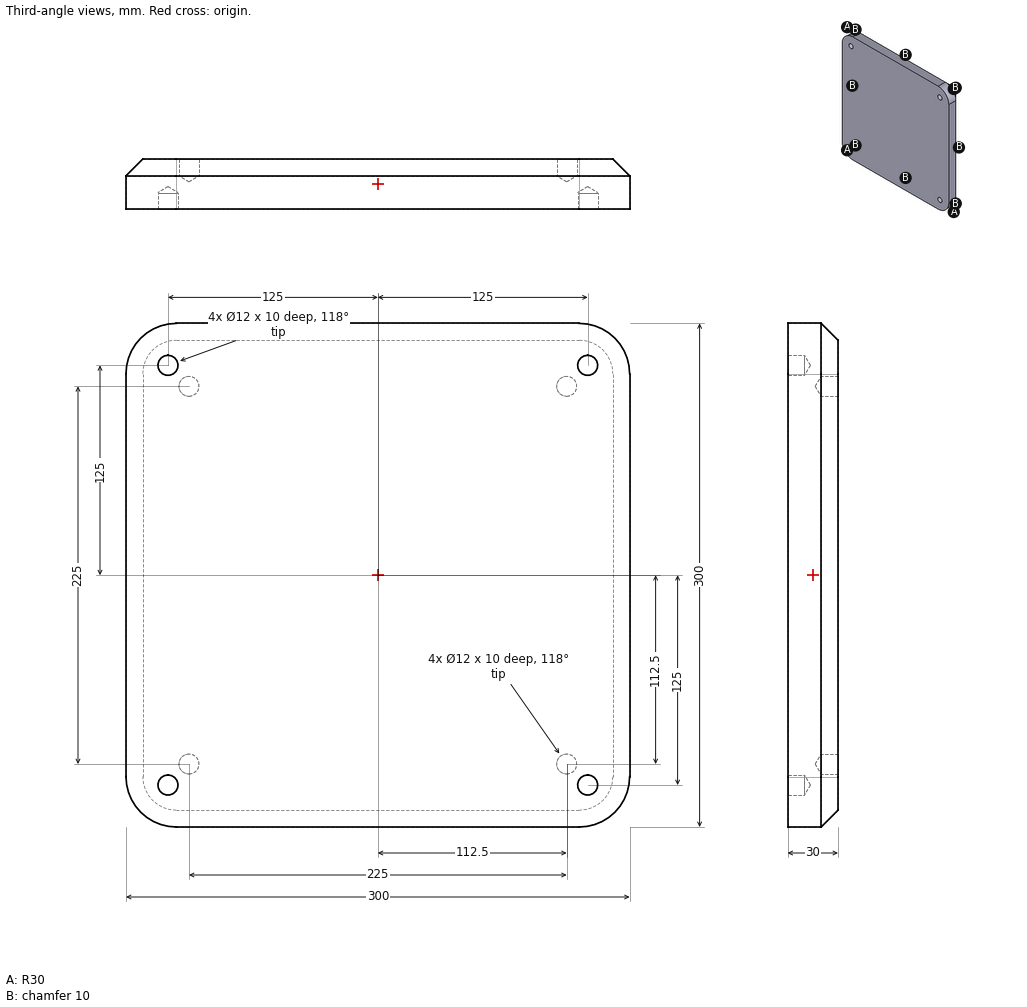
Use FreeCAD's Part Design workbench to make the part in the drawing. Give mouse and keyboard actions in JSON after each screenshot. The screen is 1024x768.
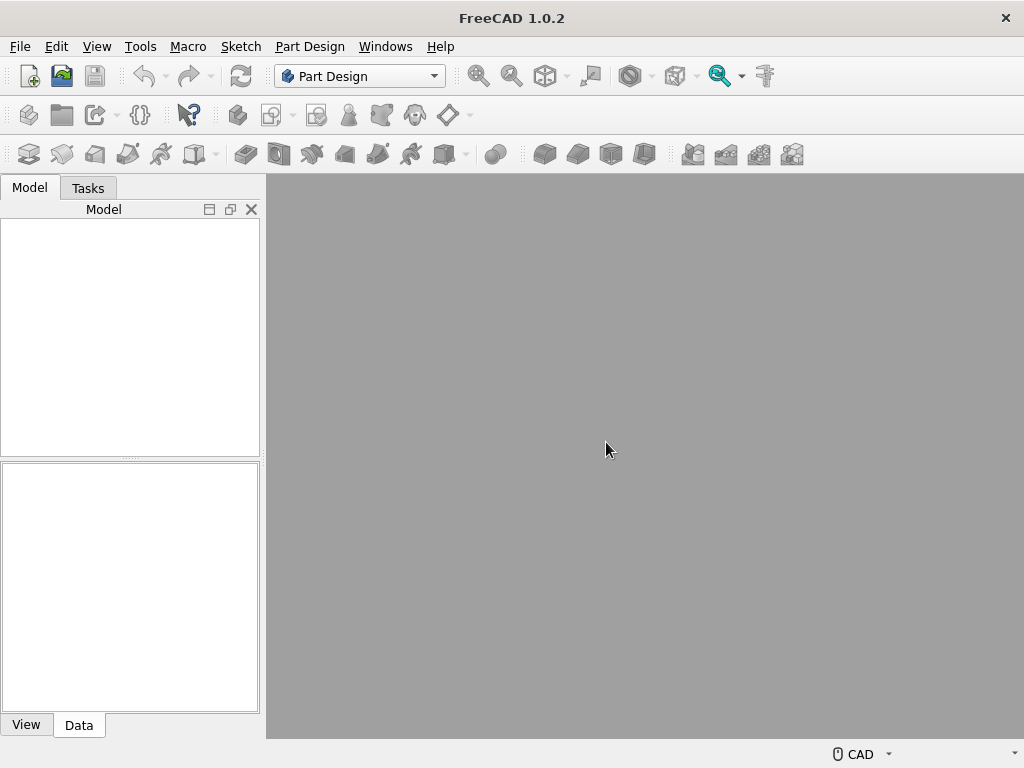
{"action": "left_click", "coordinate": [29, 76]}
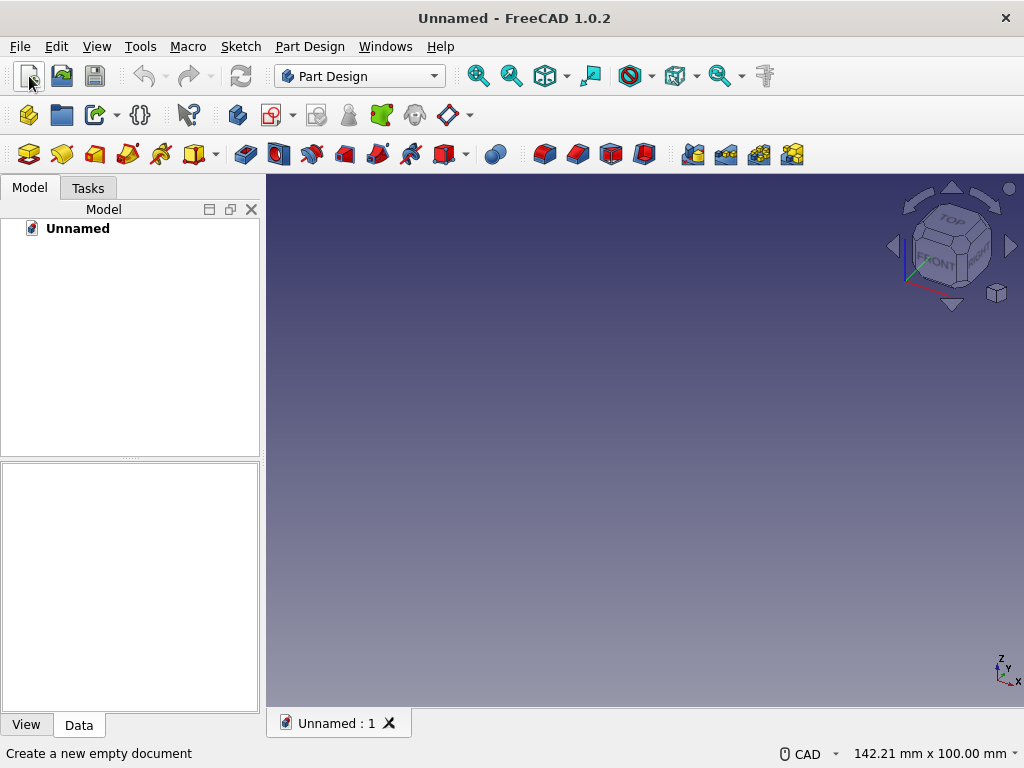
{"action": "left_click", "coordinate": [270, 116]}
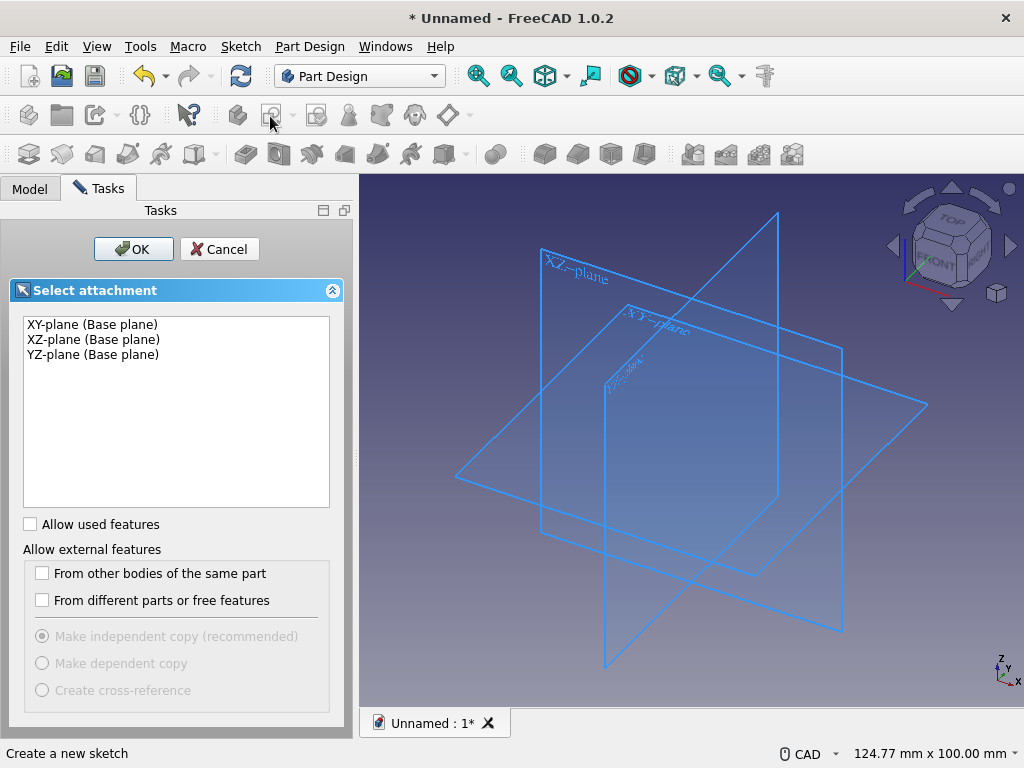
{"action": "left_click", "coordinate": [84, 340]}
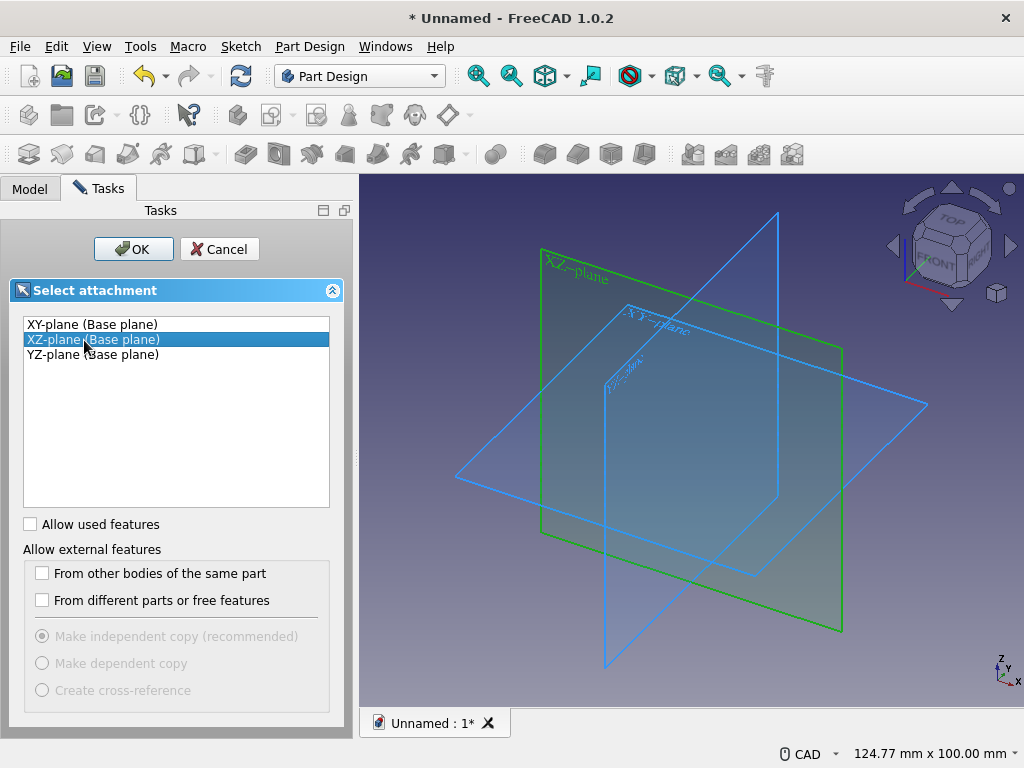
{"action": "left_click", "coordinate": [134, 249]}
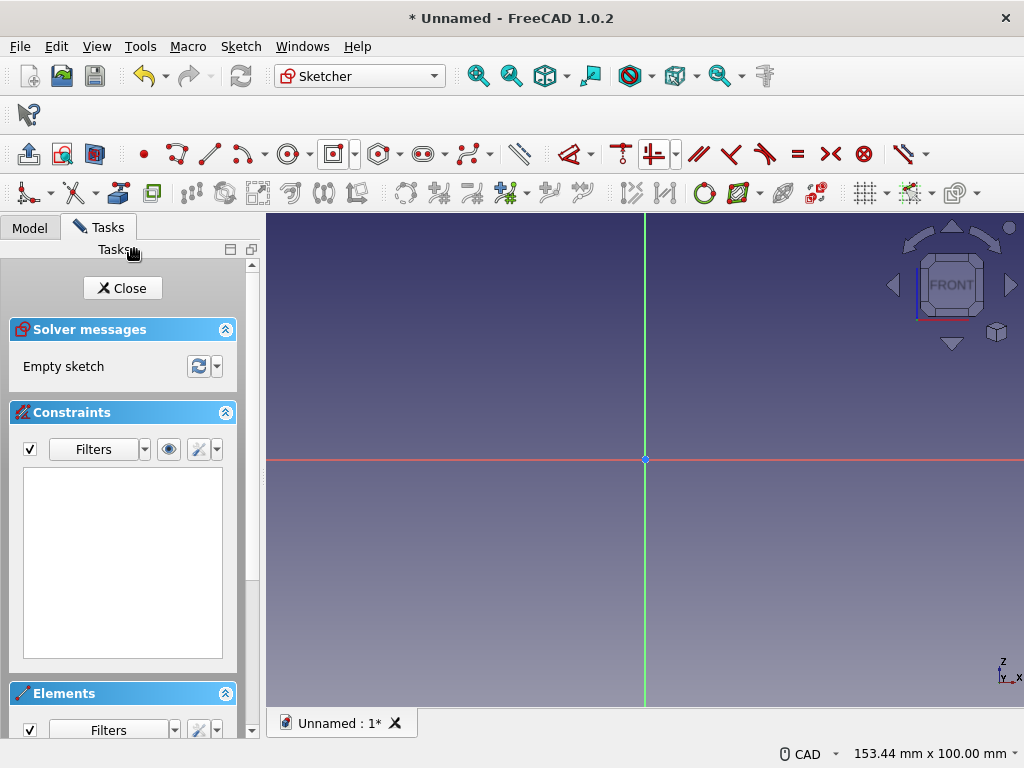
{"action": "scroll", "coordinate": [559, 460], "scroll_direction": "down", "scroll_amount": 8}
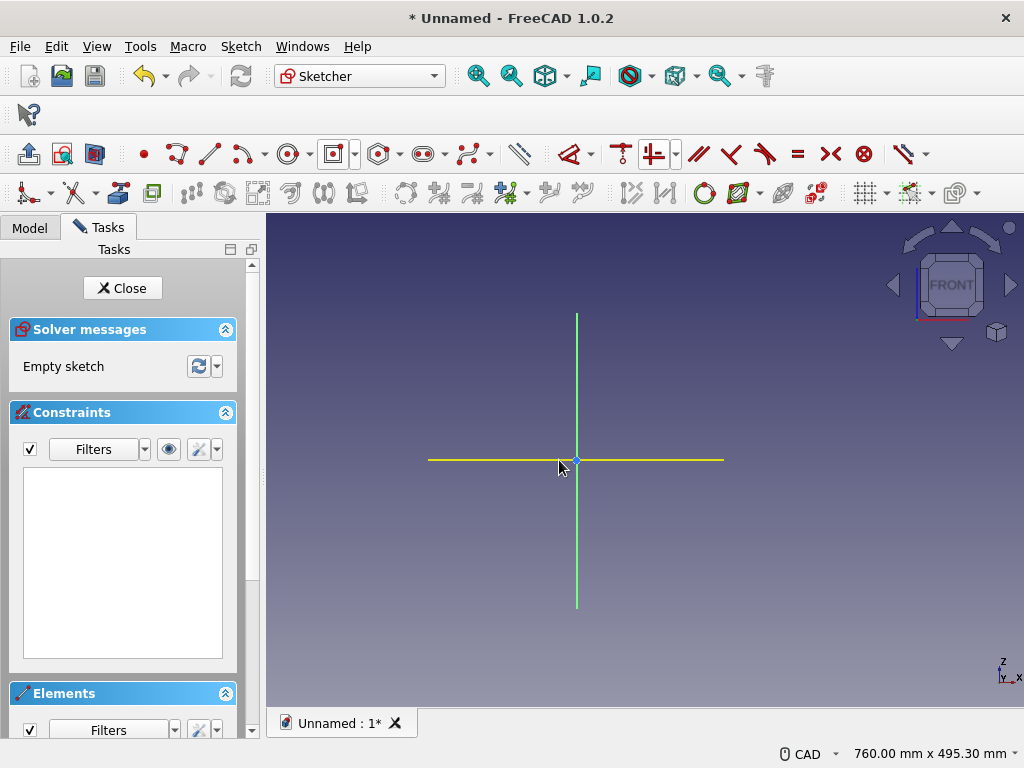
{"action": "left_click", "coordinate": [332, 154]}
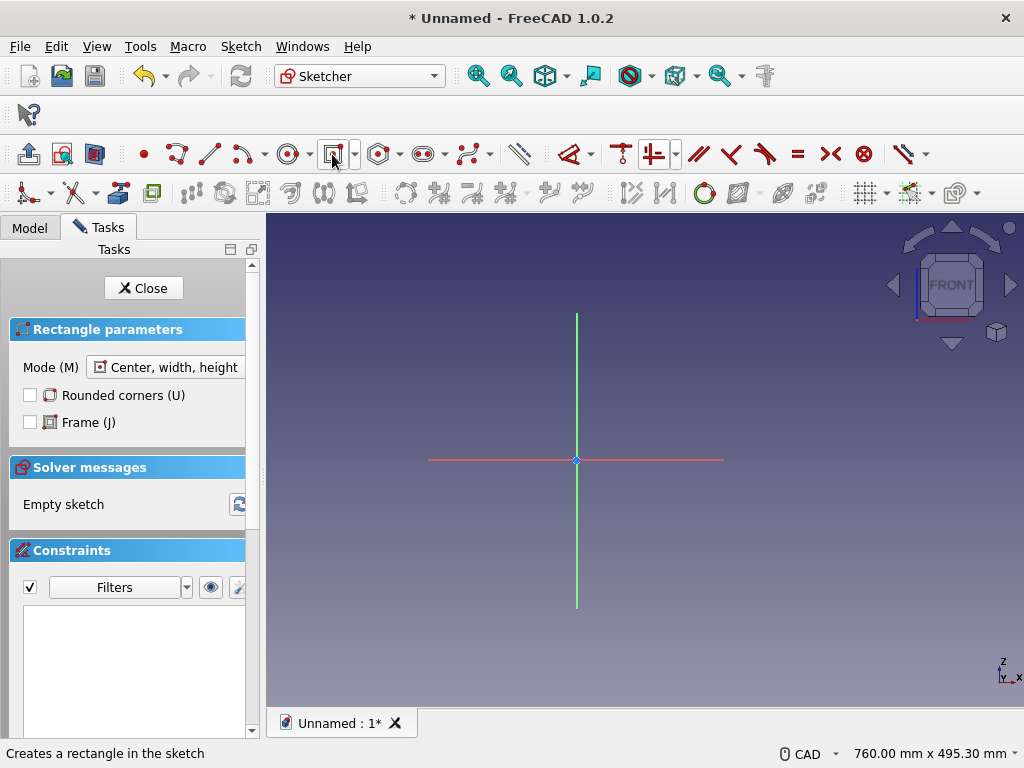
{"action": "left_click", "coordinate": [577, 460]}
{"action": "left_click", "coordinate": [726, 311]}
{"action": "key", "text": "Escape"}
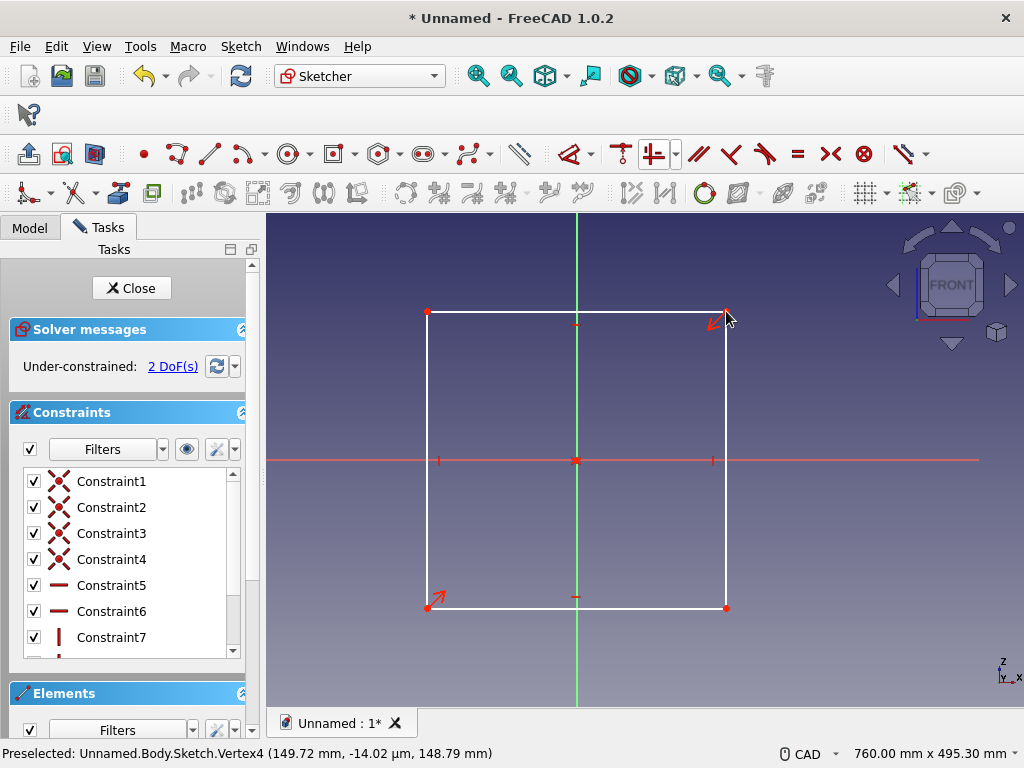
{"action": "left_click", "coordinate": [568, 154]}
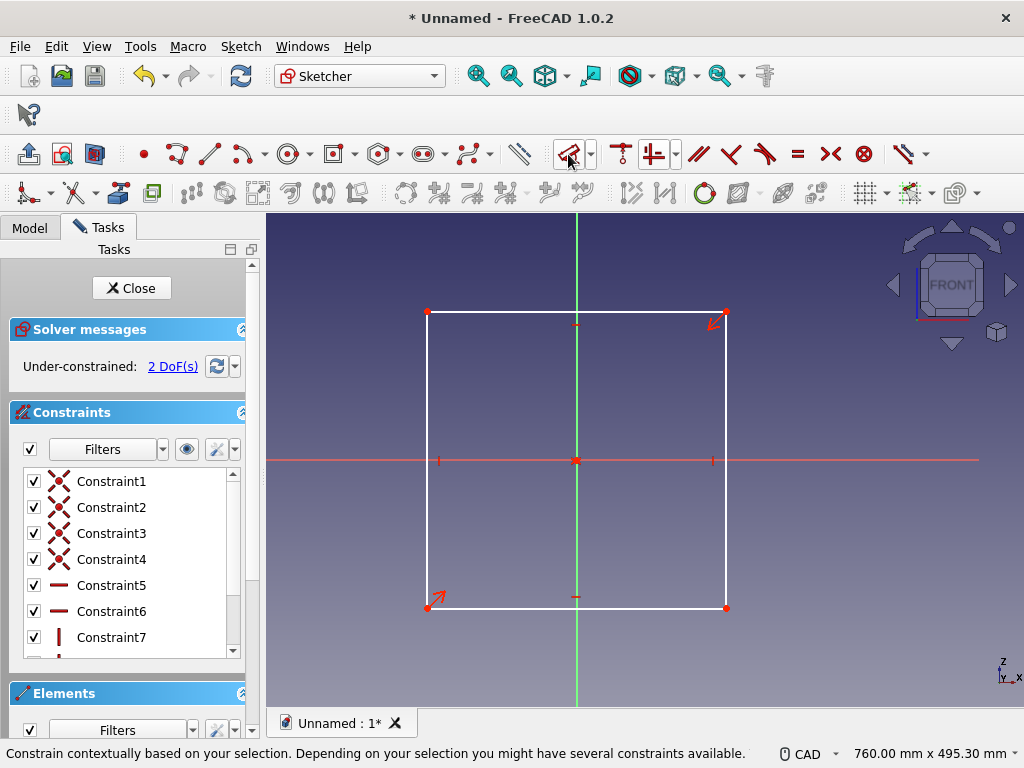
{"action": "left_click", "coordinate": [517, 609]}
{"action": "left_click", "coordinate": [508, 643]}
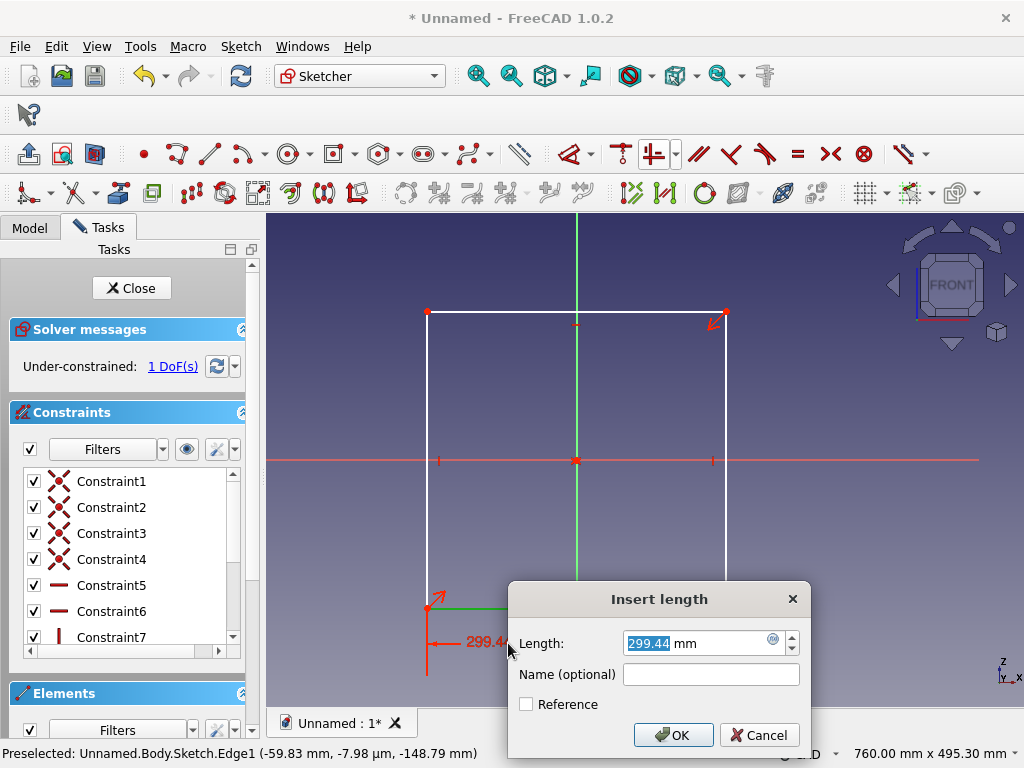
{"action": "type", "text": "300"}
{"action": "key", "text": "Return"}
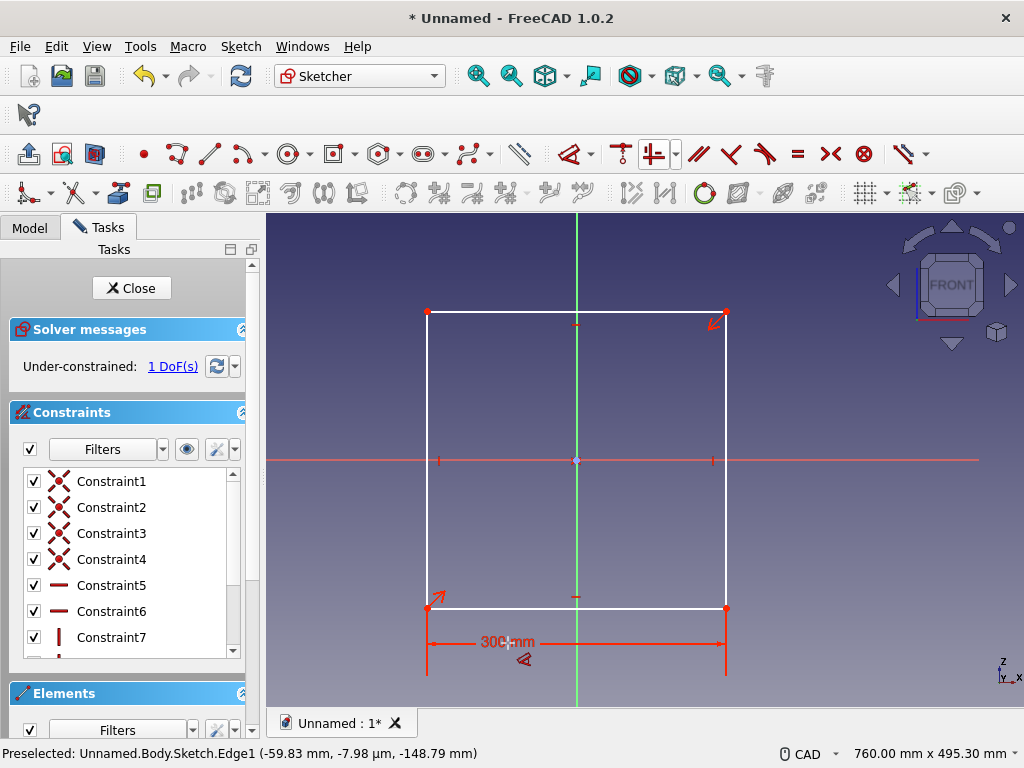
{"action": "left_click", "coordinate": [726, 520]}
{"action": "left_click", "coordinate": [760, 392]}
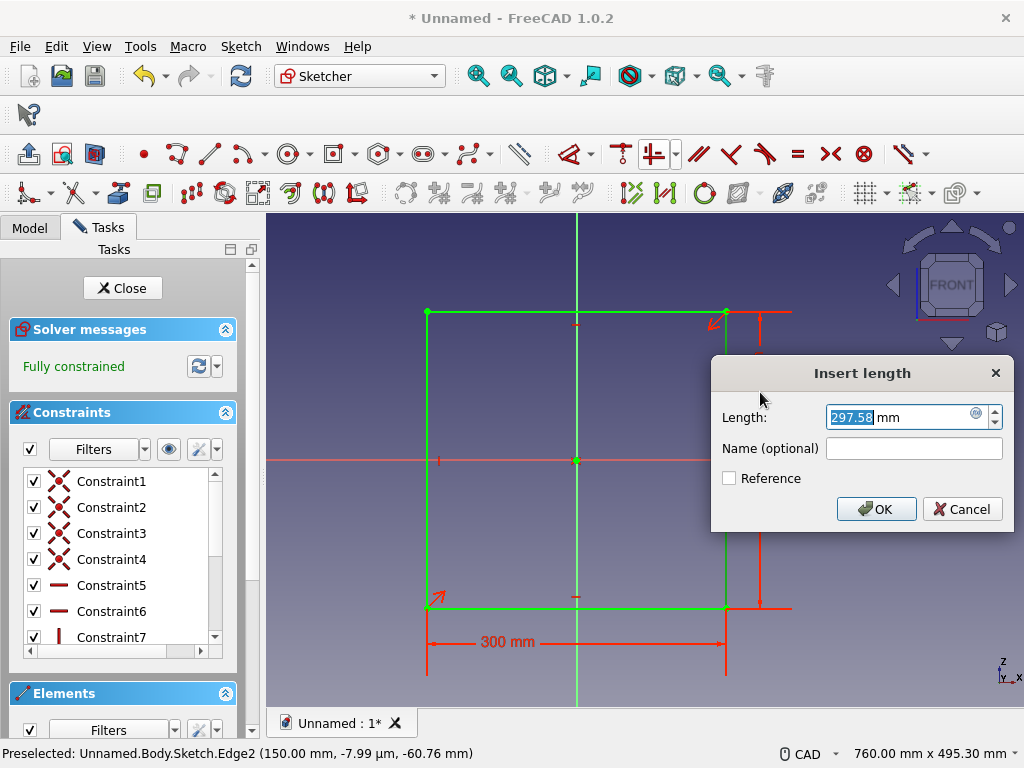
{"action": "type", "text": "300"}
{"action": "key", "text": "Return"}
{"action": "key", "text": "Escape"}